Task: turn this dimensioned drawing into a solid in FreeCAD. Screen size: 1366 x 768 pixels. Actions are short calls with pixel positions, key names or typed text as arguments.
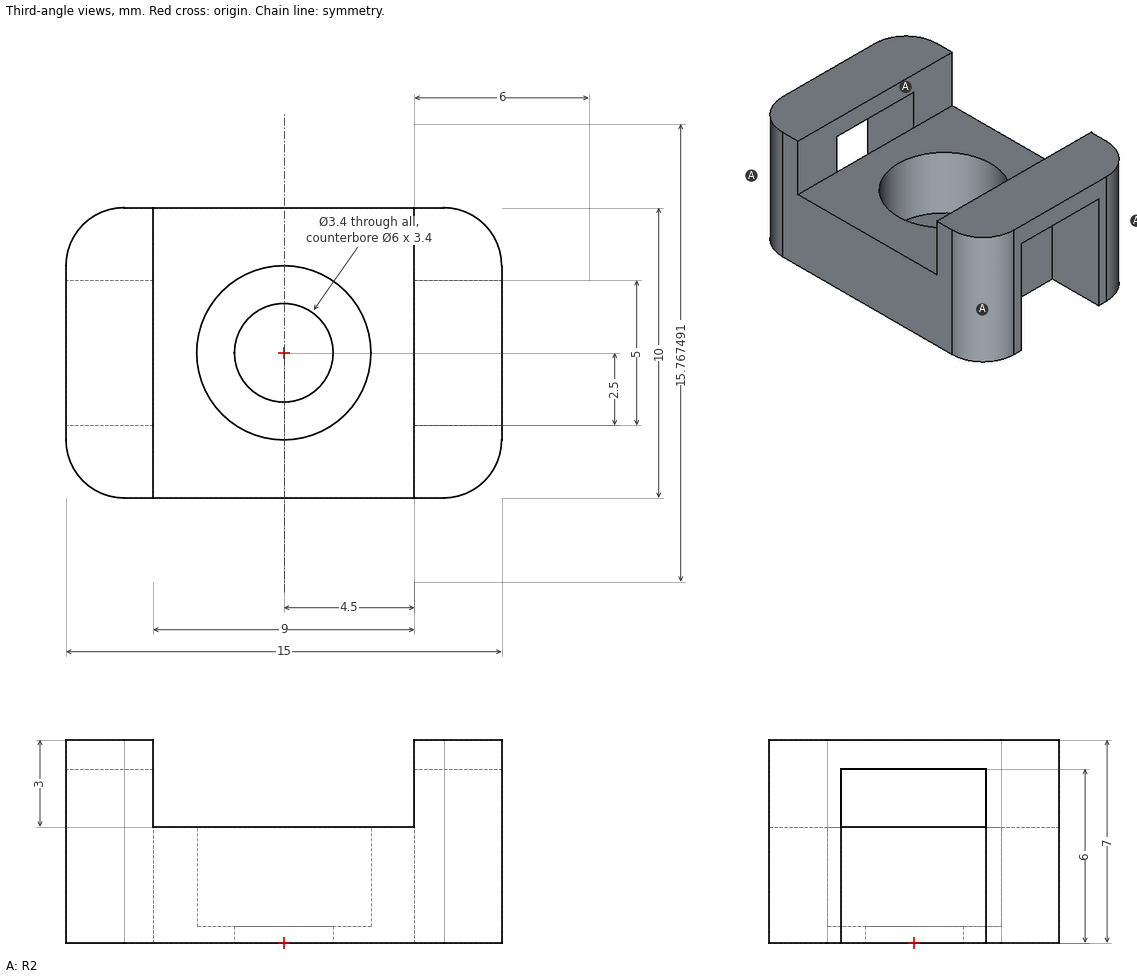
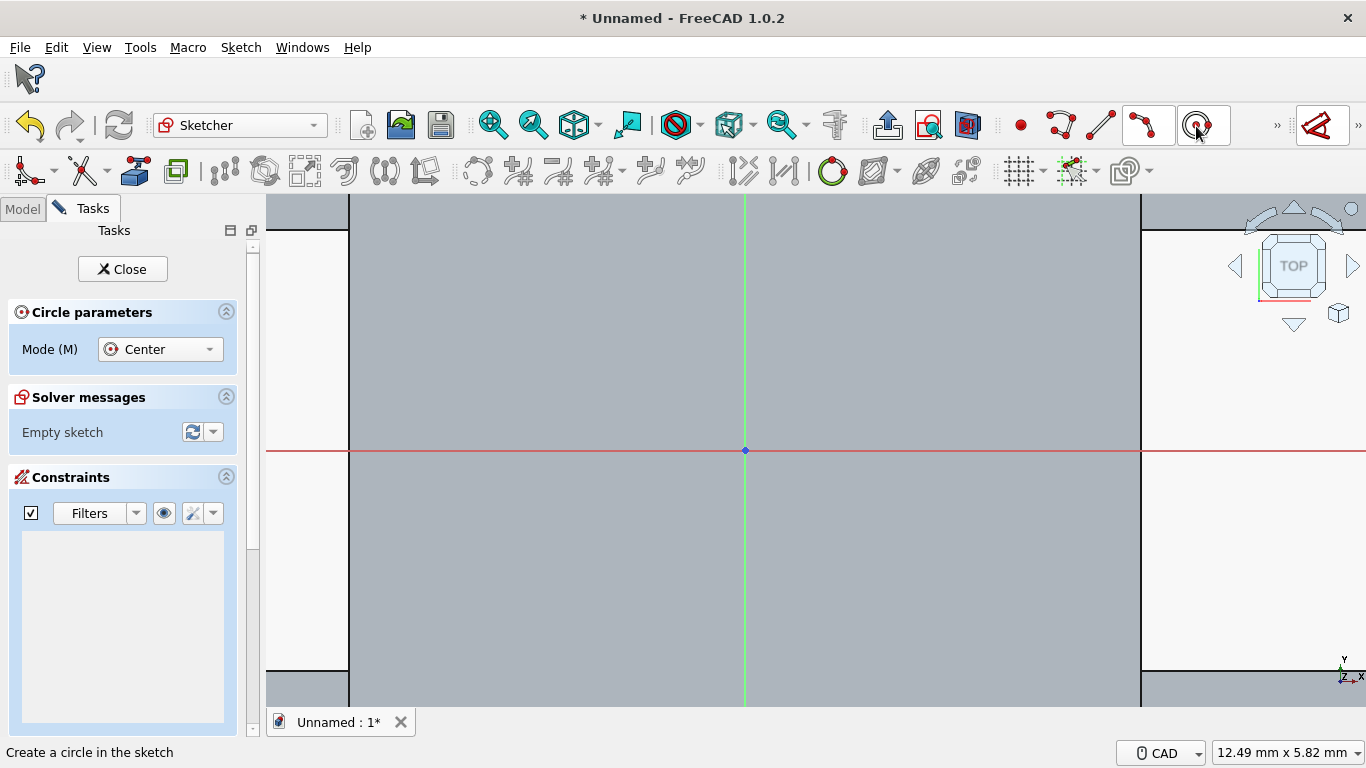
click(745, 450)
click(851, 345)
key(Escape)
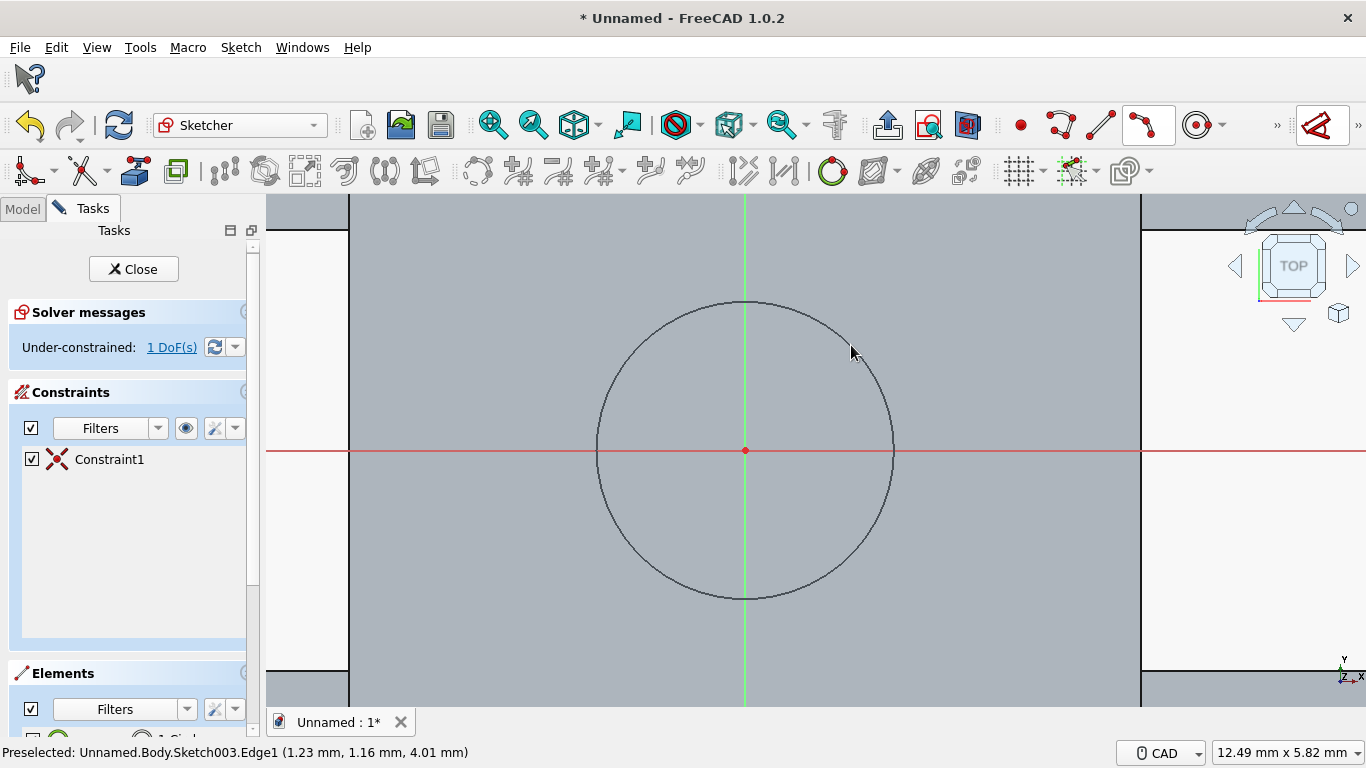
click(850, 345)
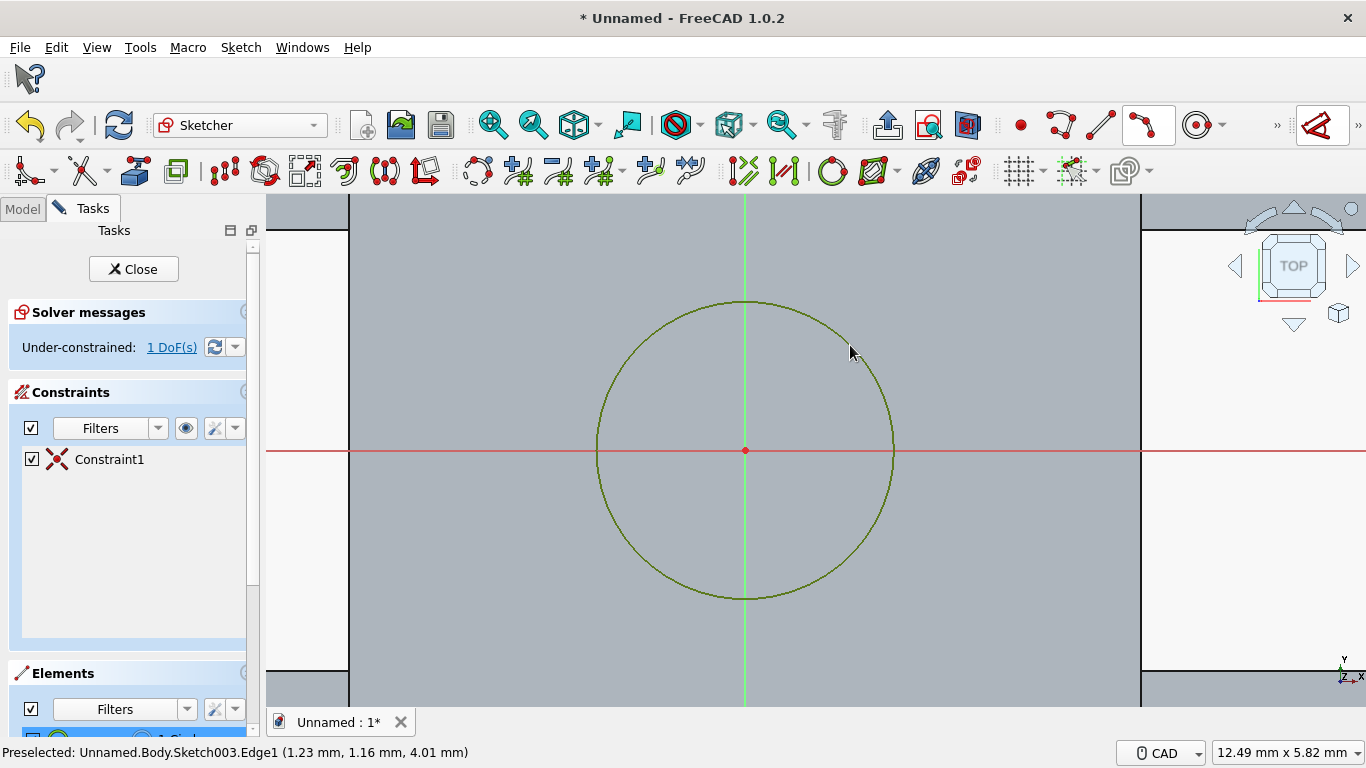
click(1344, 126)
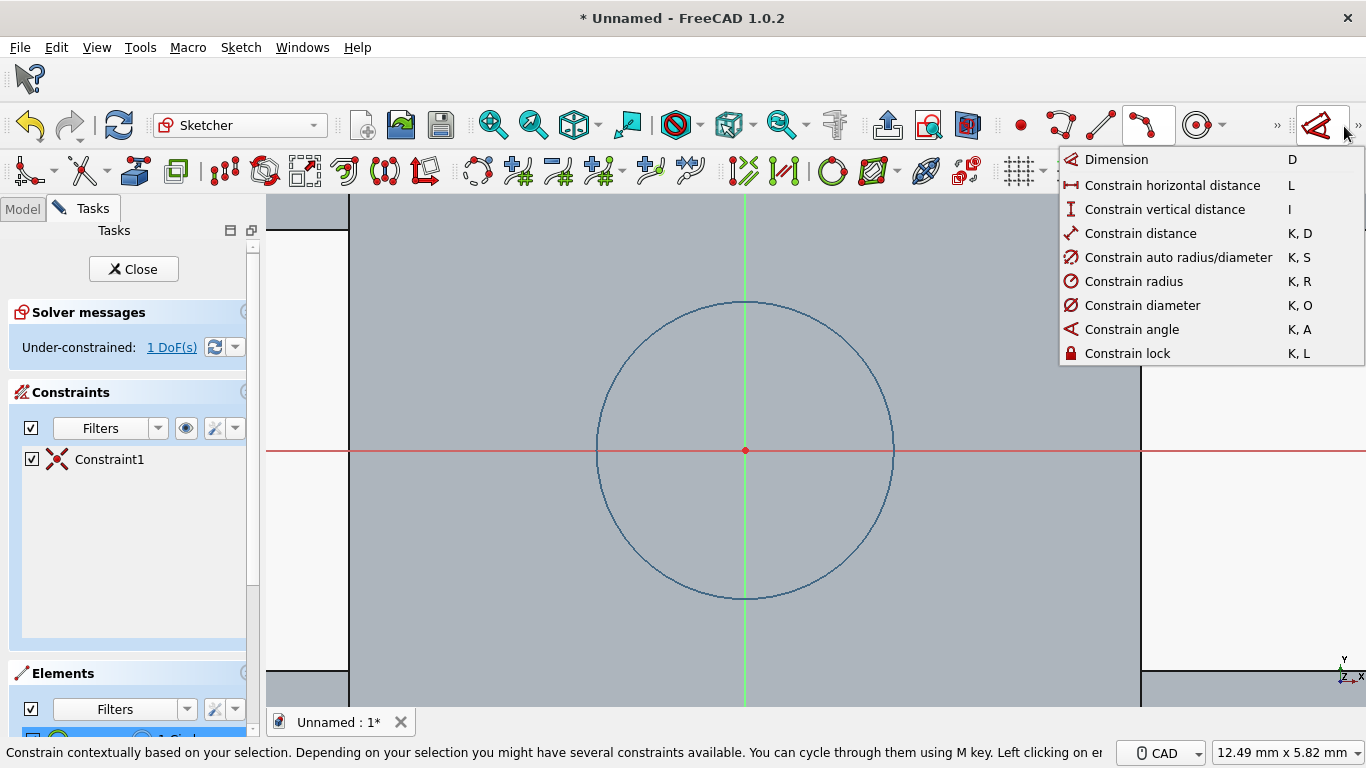
click(1212, 305)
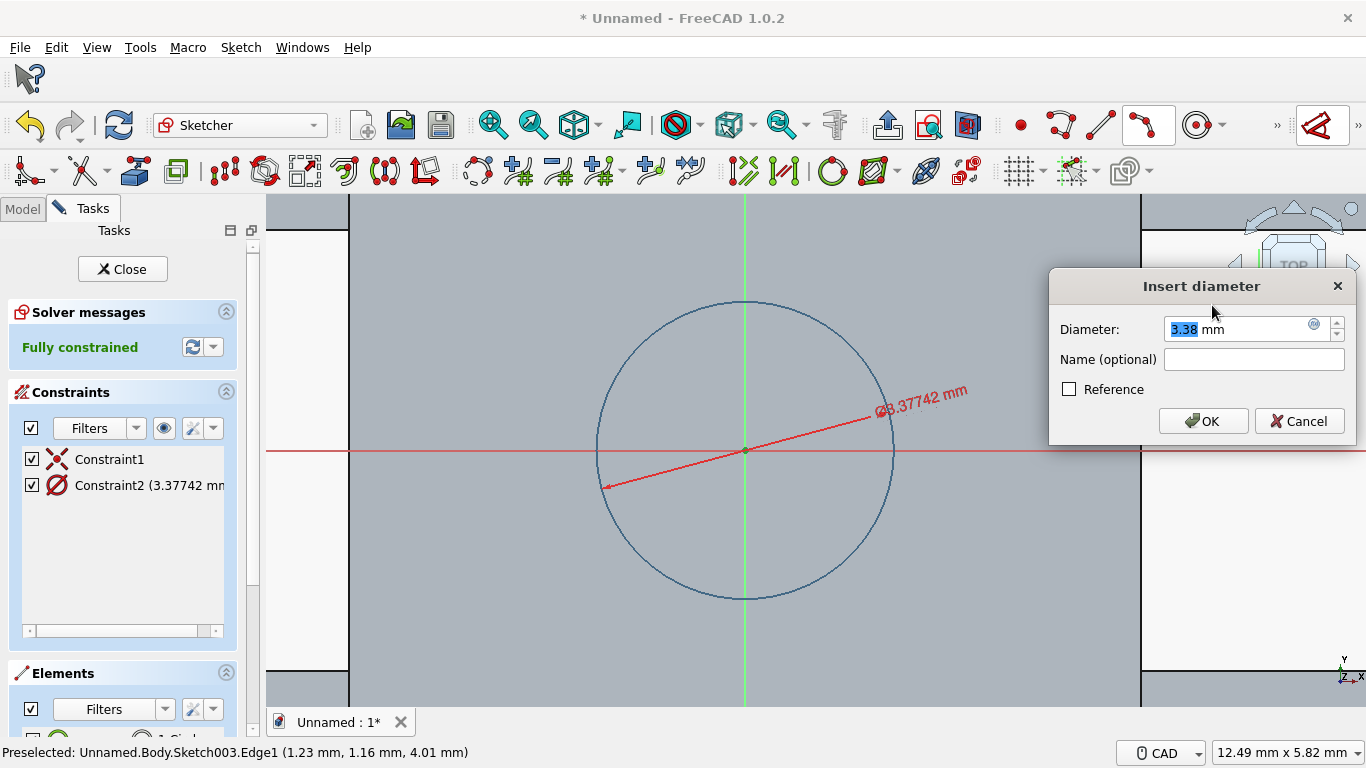
text(3.4)
key(Return)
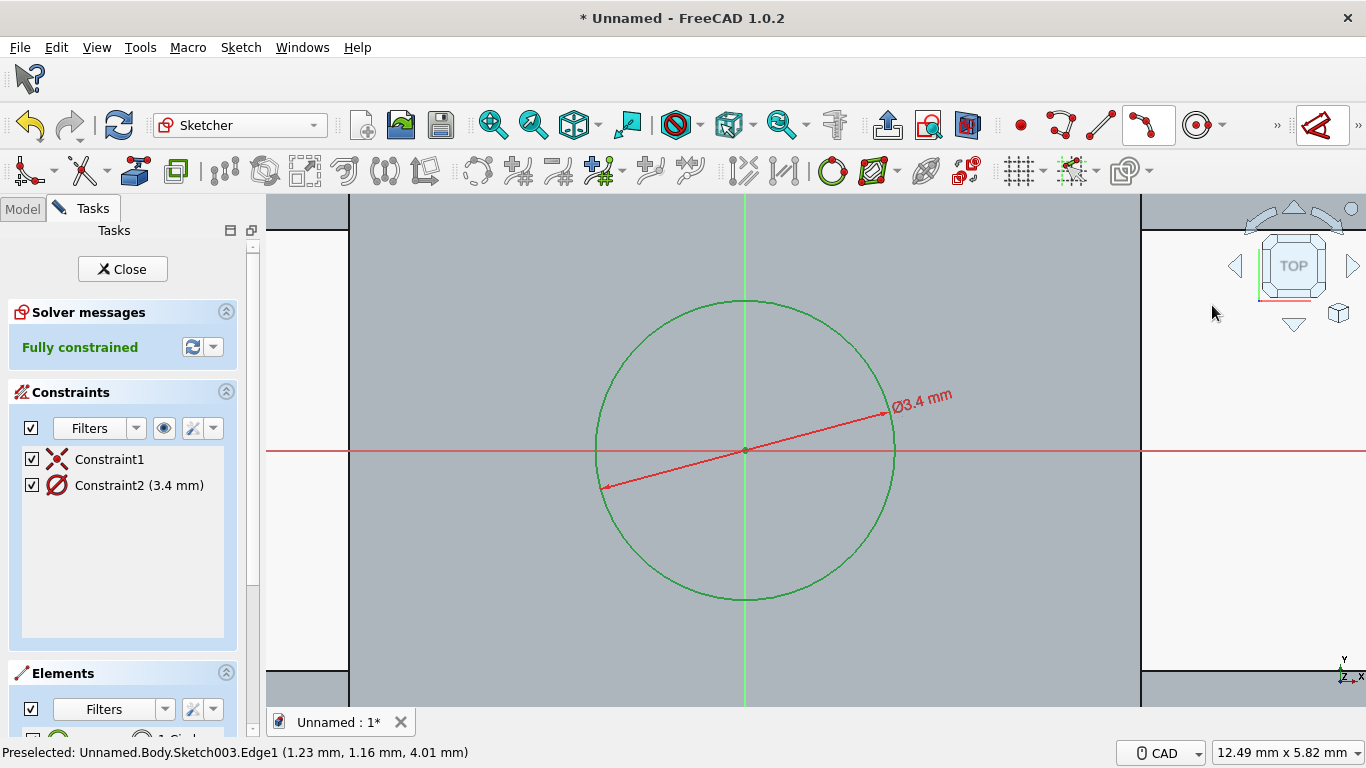
click(123, 269)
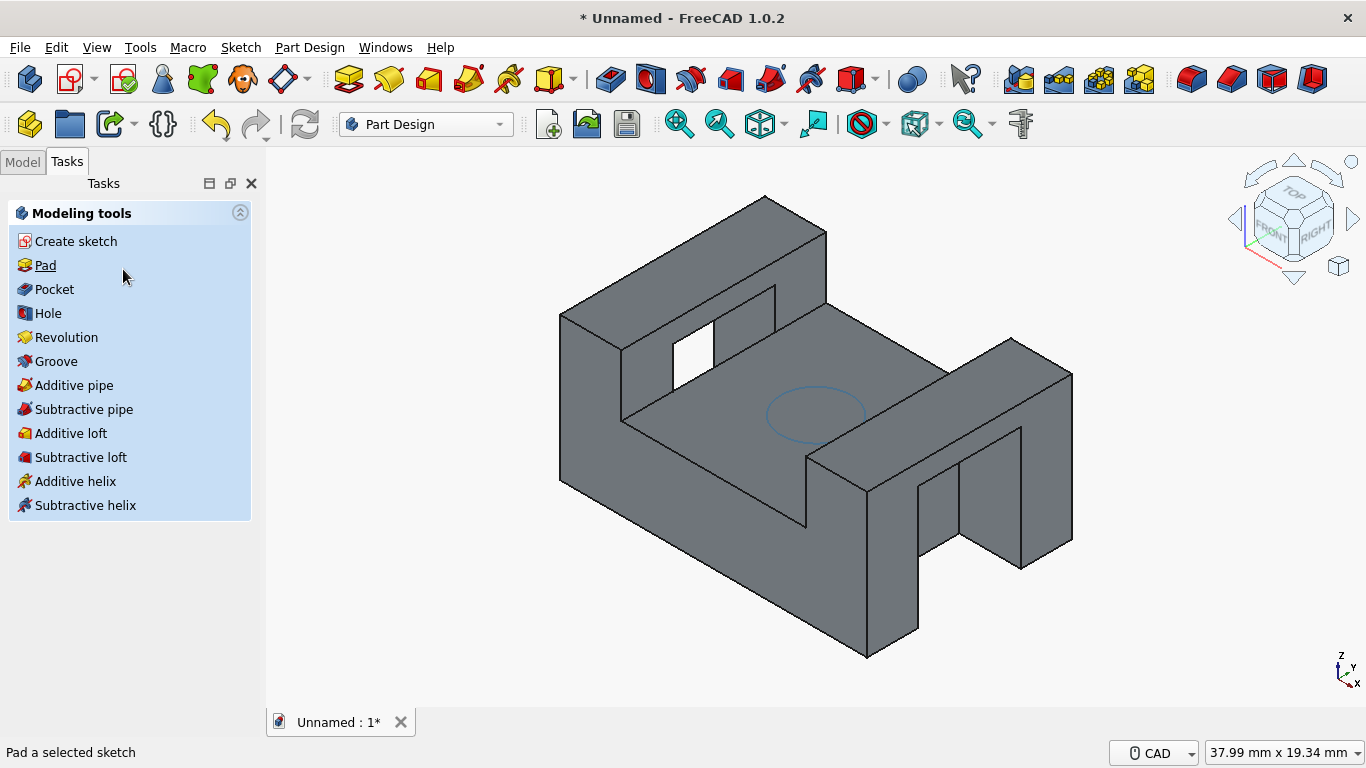
click(652, 80)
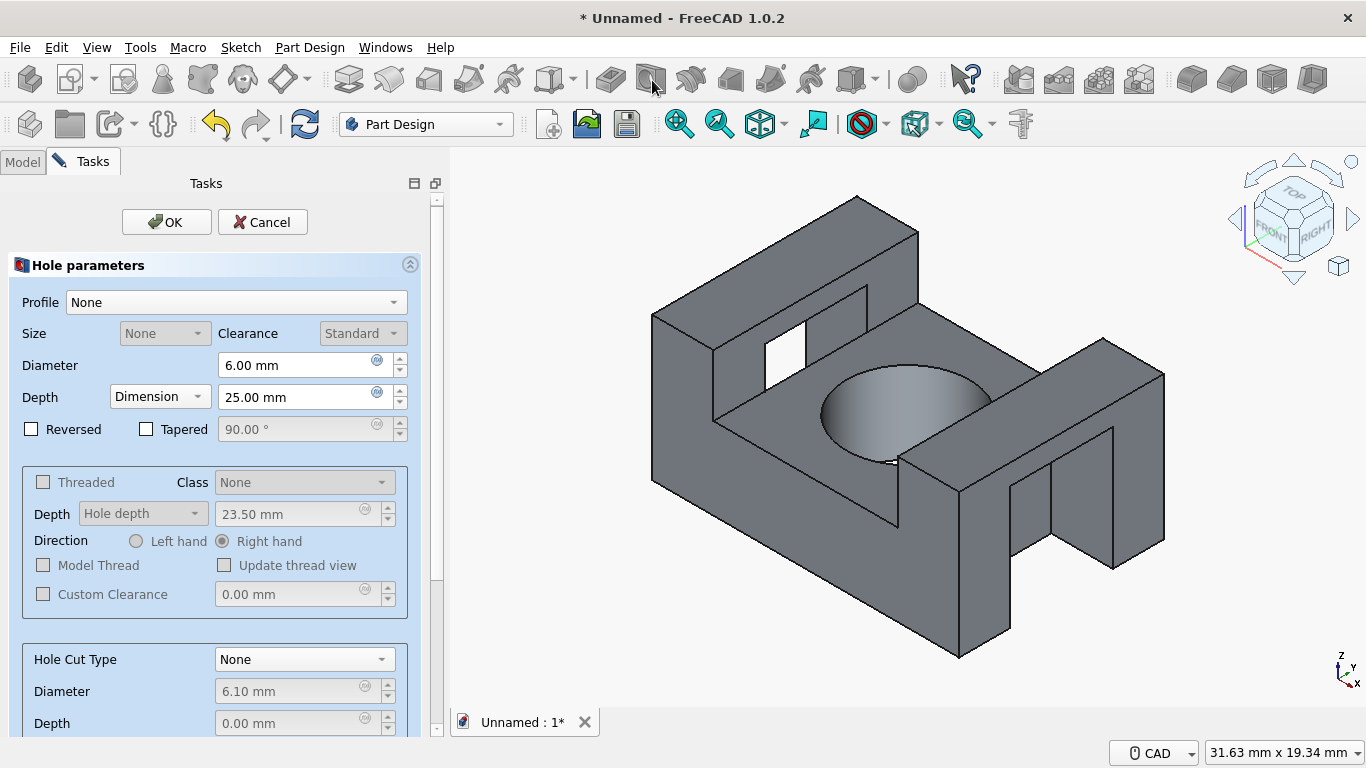
triple_click(305, 365)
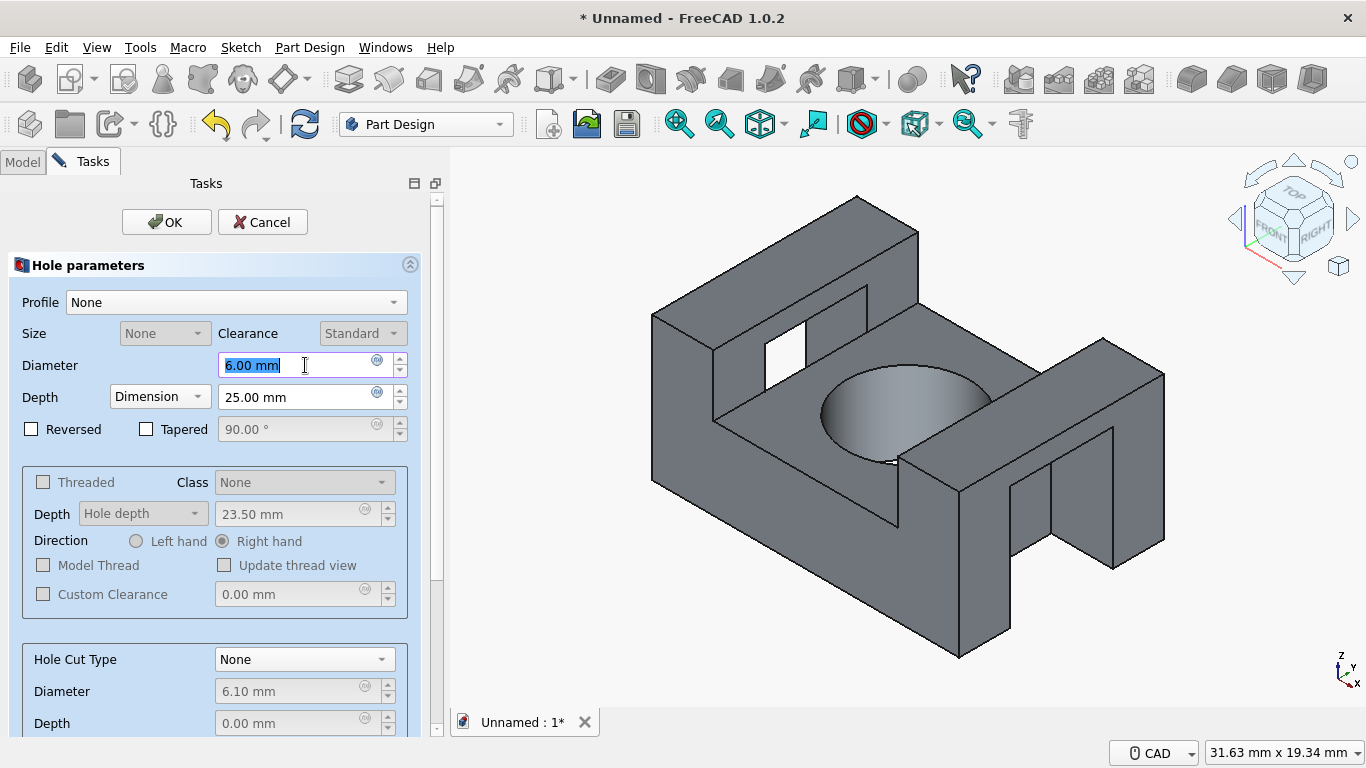
text(3.4)
key(Tab)